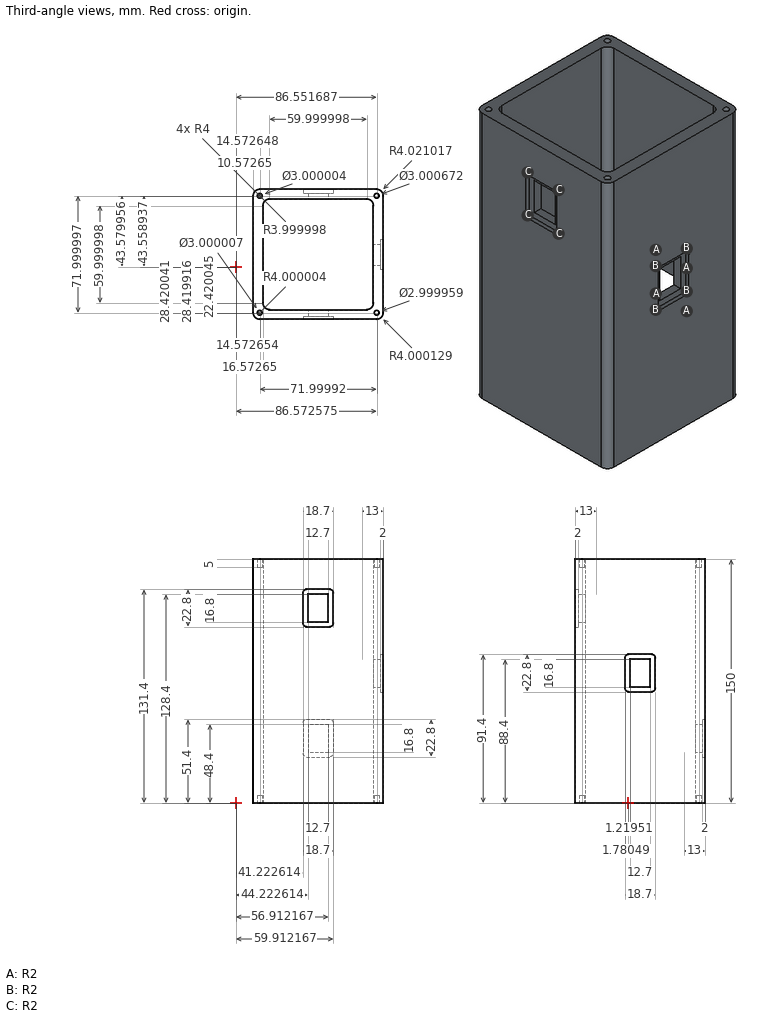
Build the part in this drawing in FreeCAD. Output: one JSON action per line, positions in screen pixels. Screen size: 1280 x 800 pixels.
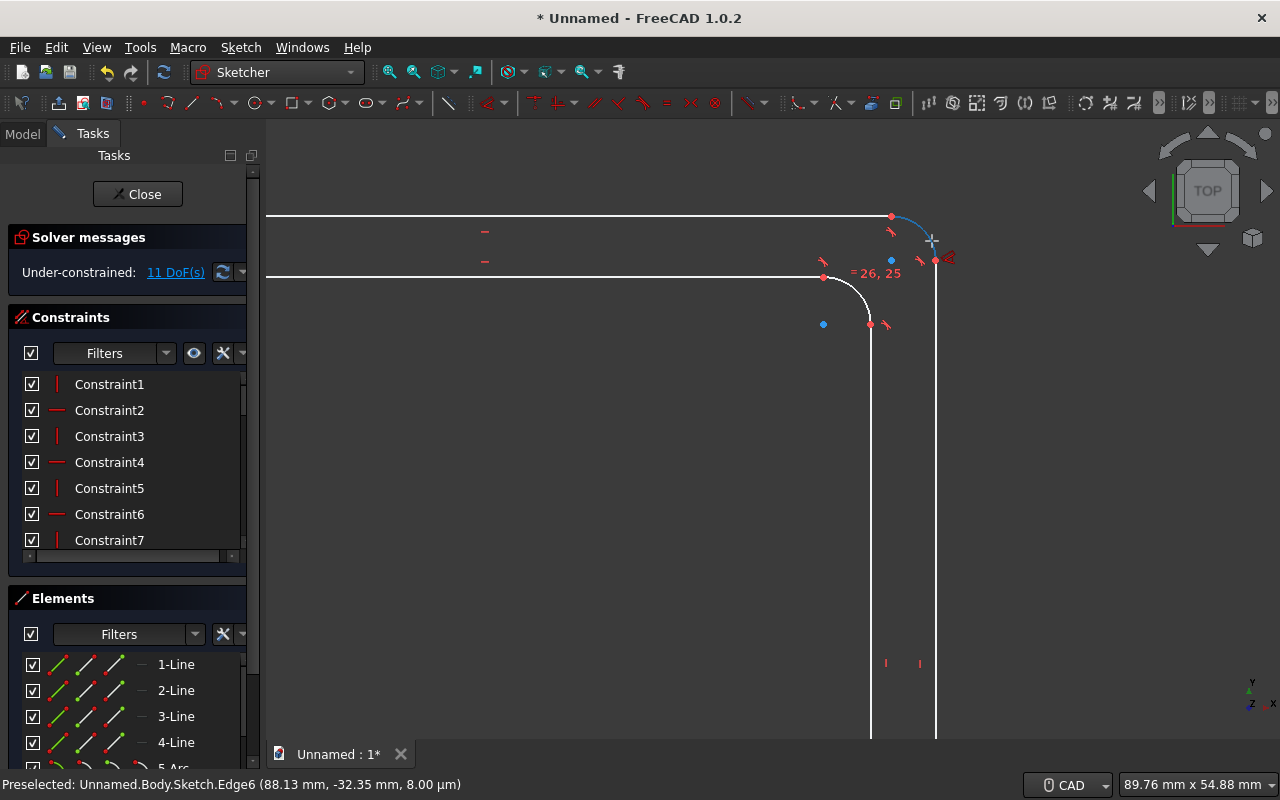
{"action": "left_click", "coordinate": [931, 241]}
{"action": "left_click", "coordinate": [960, 227]}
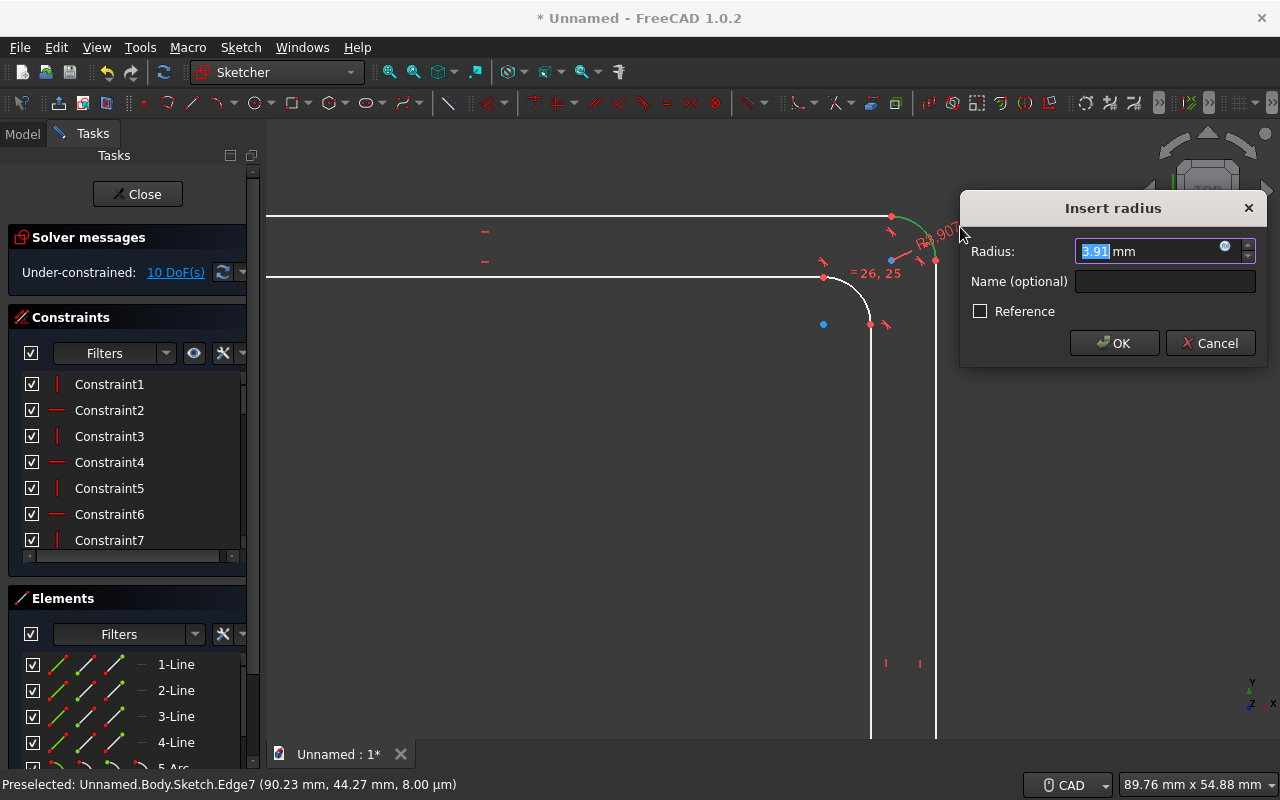
{"action": "type", "text": "4.021017"}
{"action": "key", "text": "Return"}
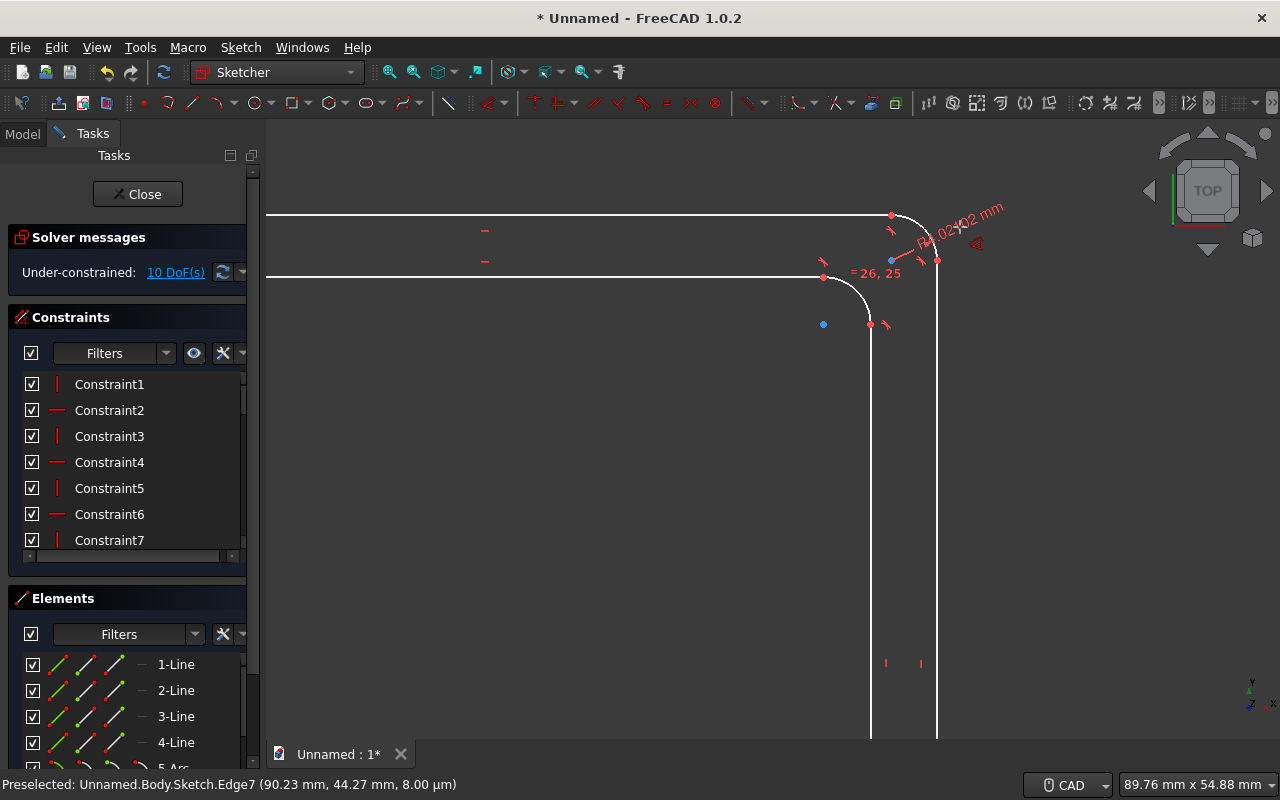
{"action": "scroll", "coordinate": [932, 240], "scroll_direction": "down", "scroll_amount": 4}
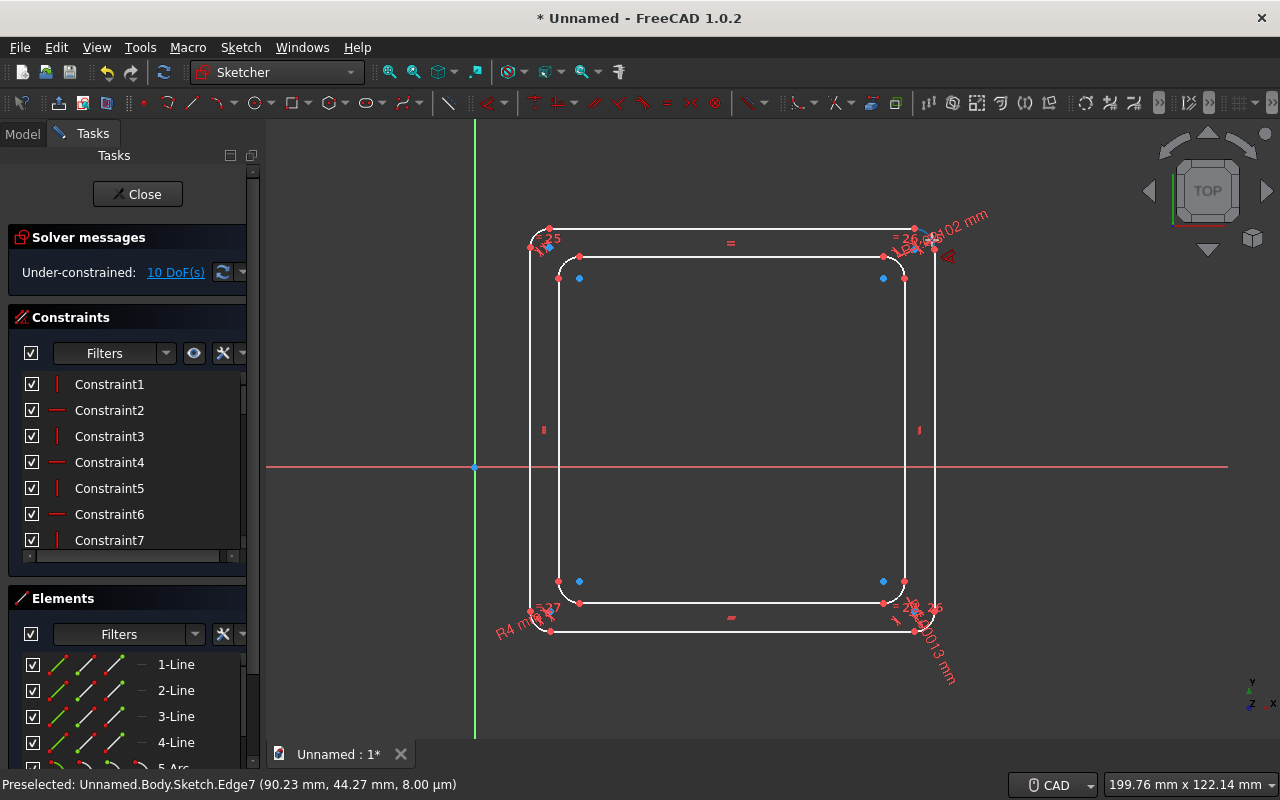
{"action": "scroll", "coordinate": [541, 231], "scroll_direction": "up", "scroll_amount": 4}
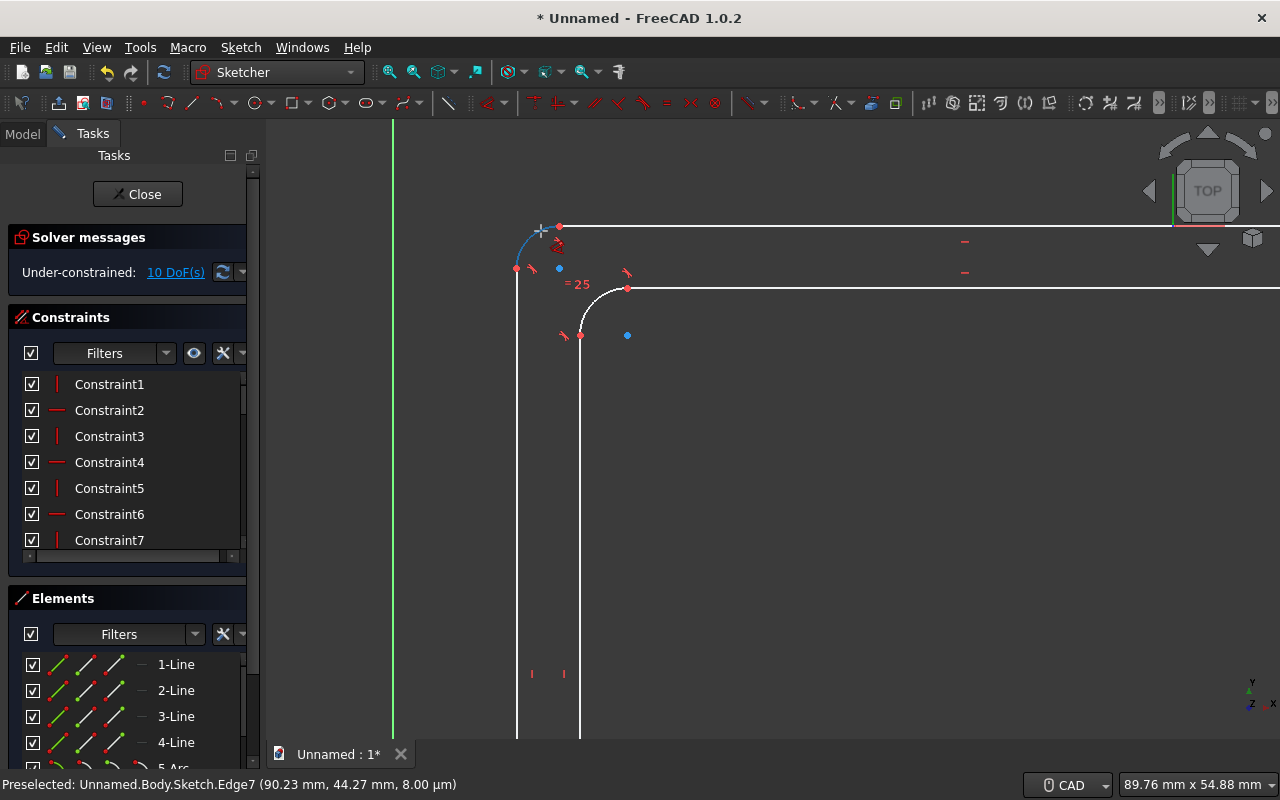
{"action": "left_click", "coordinate": [540, 231]}
{"action": "left_click", "coordinate": [526, 202]}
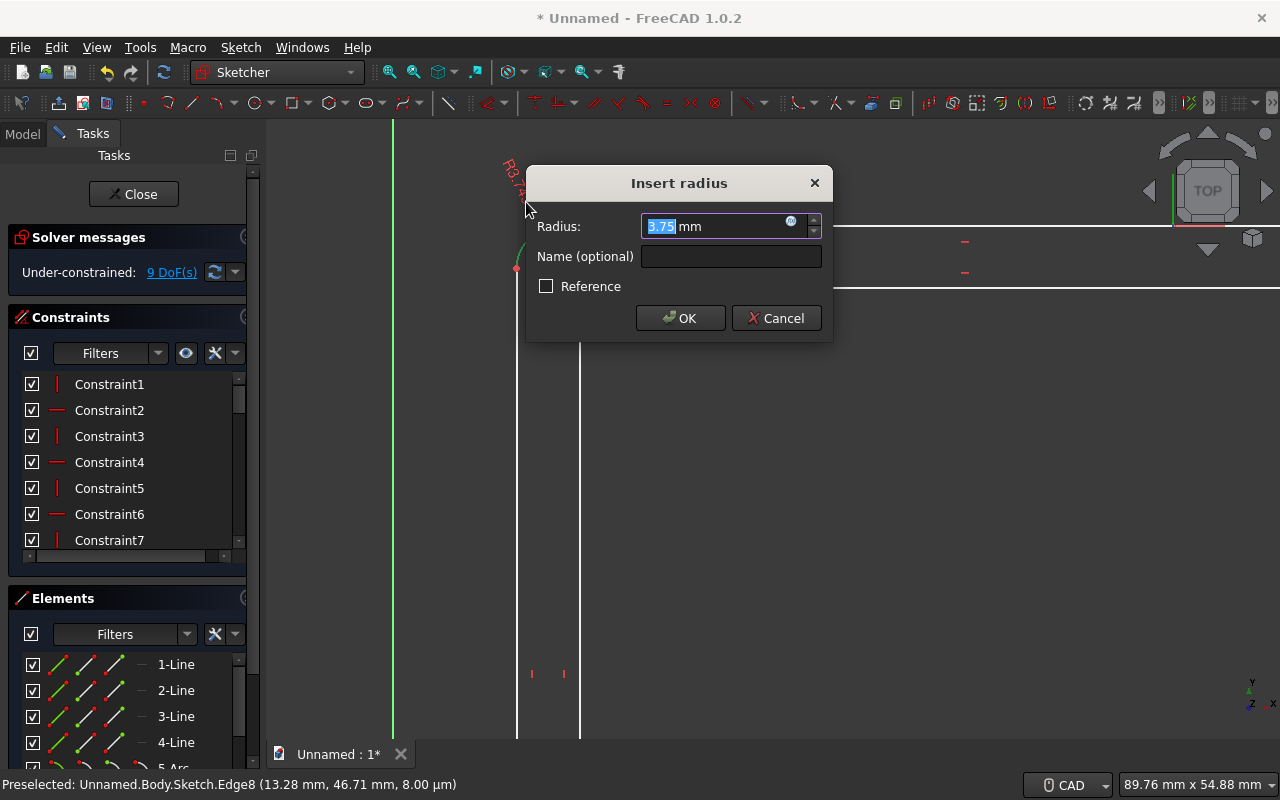
{"action": "type", "text": "3.999998"}
{"action": "key", "text": "Return"}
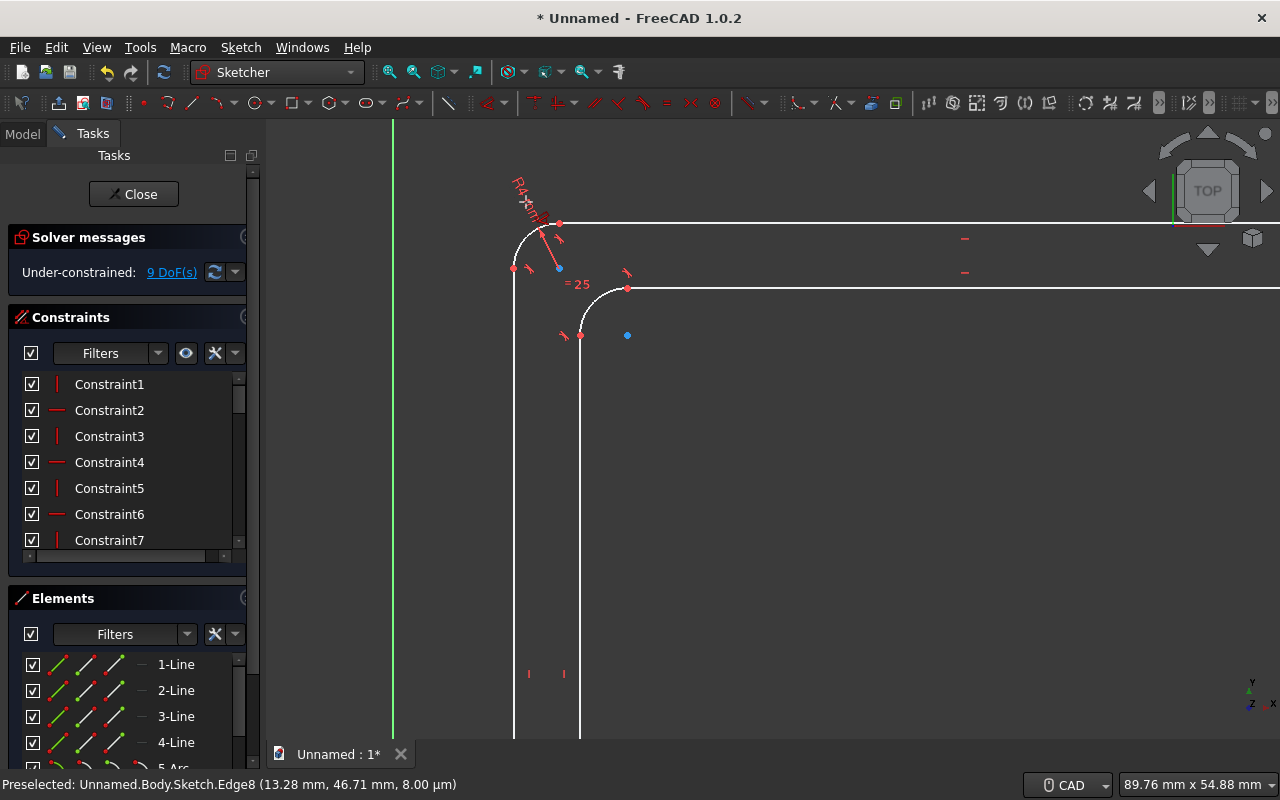
{"action": "left_click", "coordinate": [606, 293]}
{"action": "left_click", "coordinate": [592, 264]}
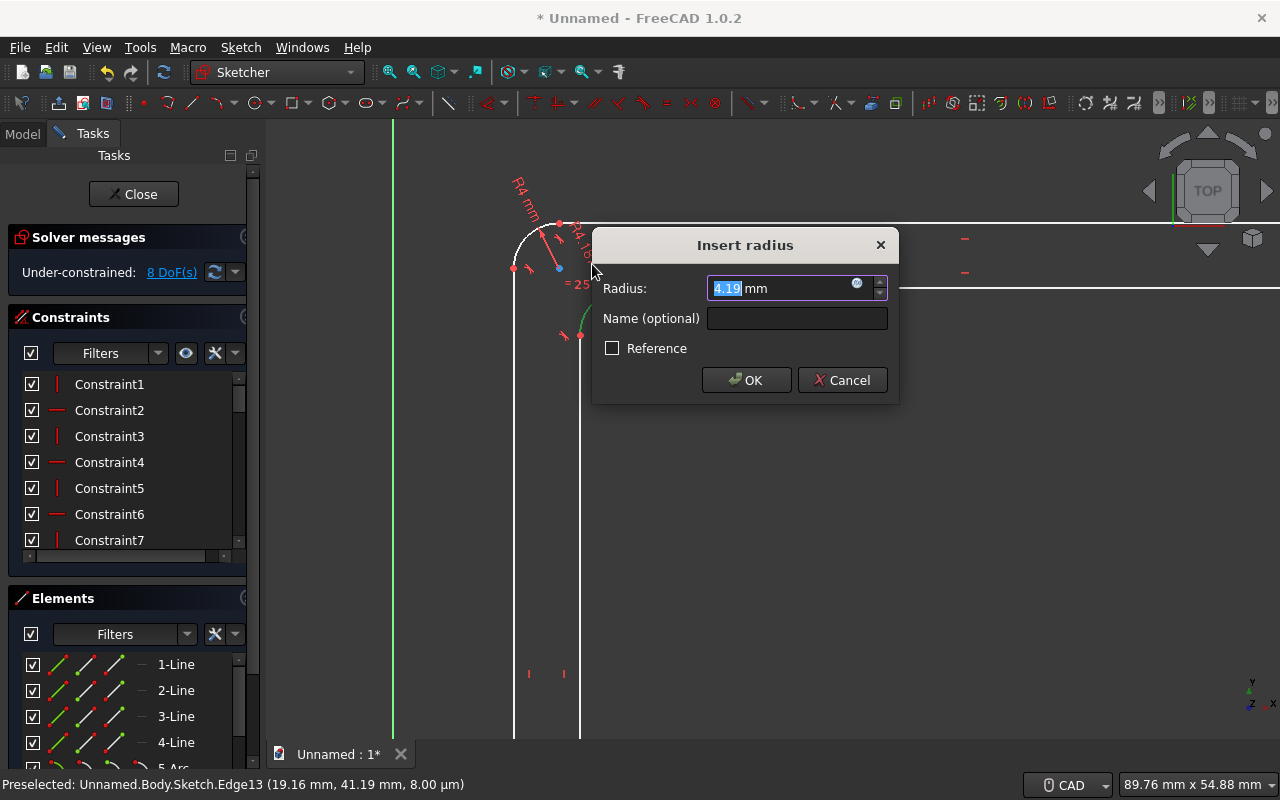
{"action": "type", "text": "4"}
{"action": "key", "text": "Return"}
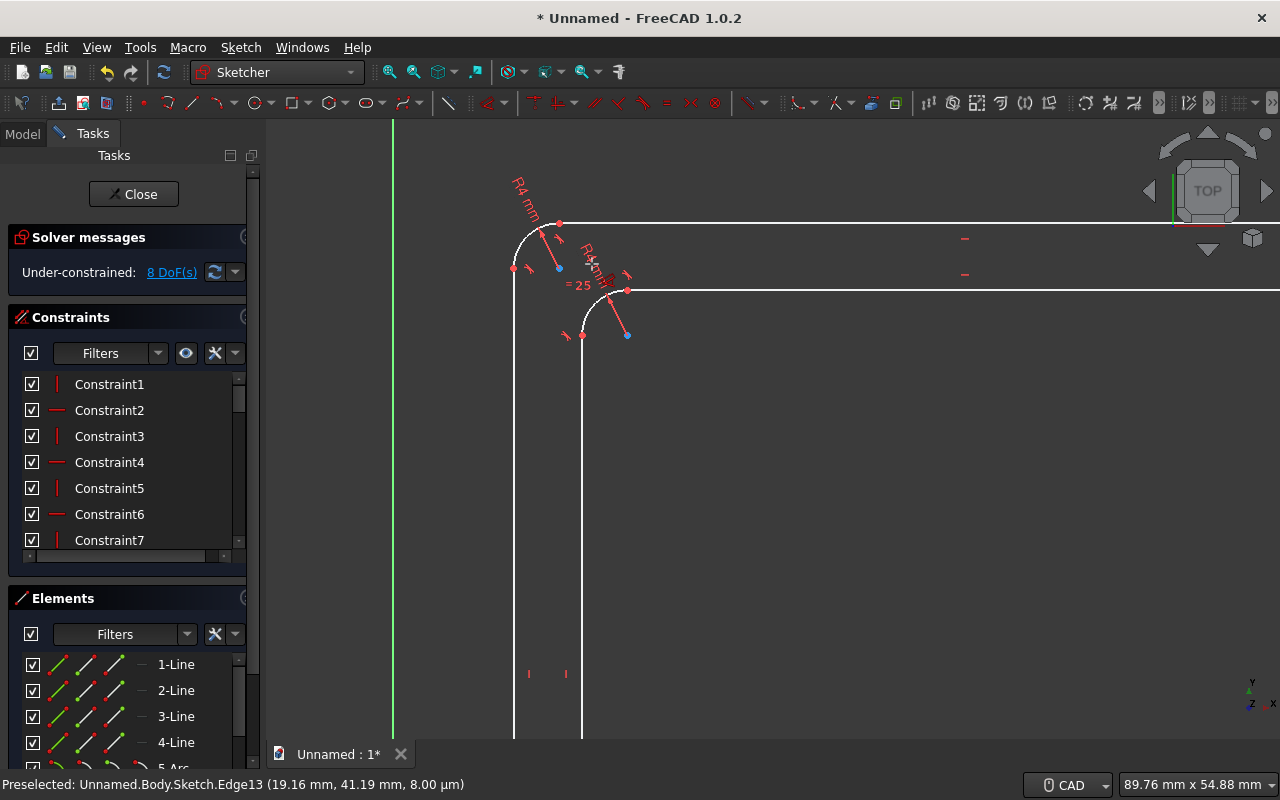
{"action": "scroll", "coordinate": [541, 231], "scroll_direction": "down", "scroll_amount": 4}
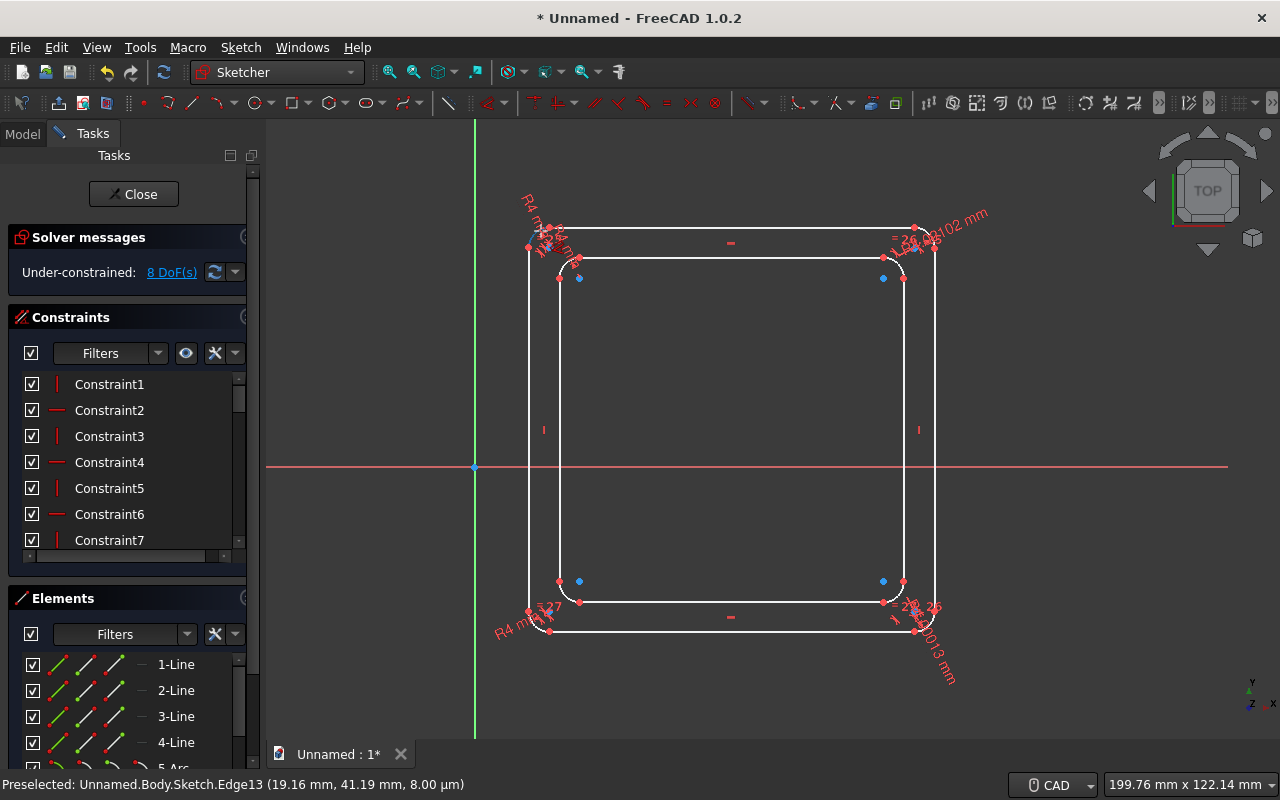
{"action": "left_click", "coordinate": [659, 632]}
{"action": "left_click", "coordinate": [732, 666]}